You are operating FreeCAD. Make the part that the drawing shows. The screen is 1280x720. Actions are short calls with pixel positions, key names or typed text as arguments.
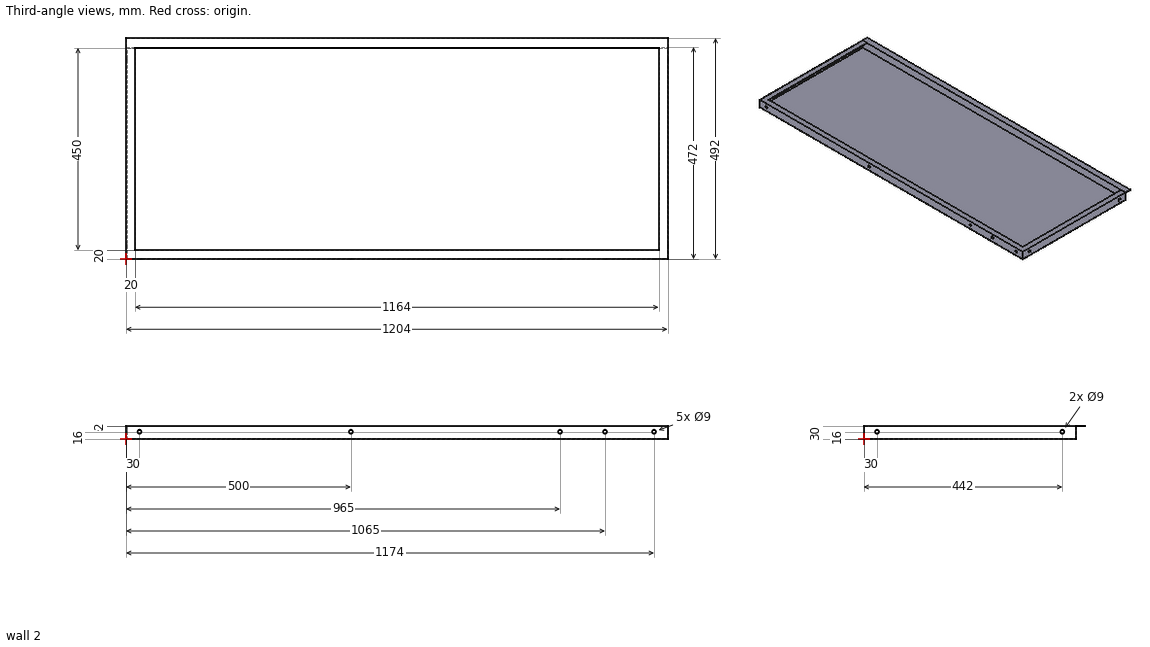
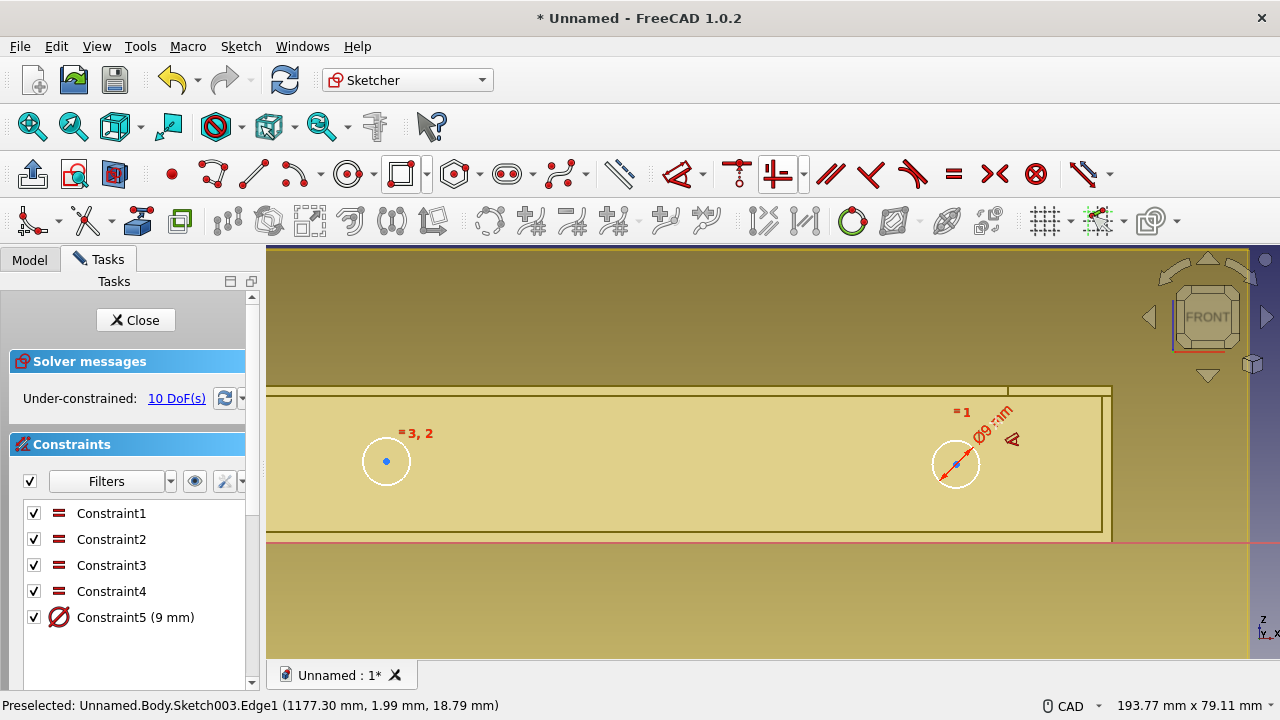
click(956, 464)
click(990, 503)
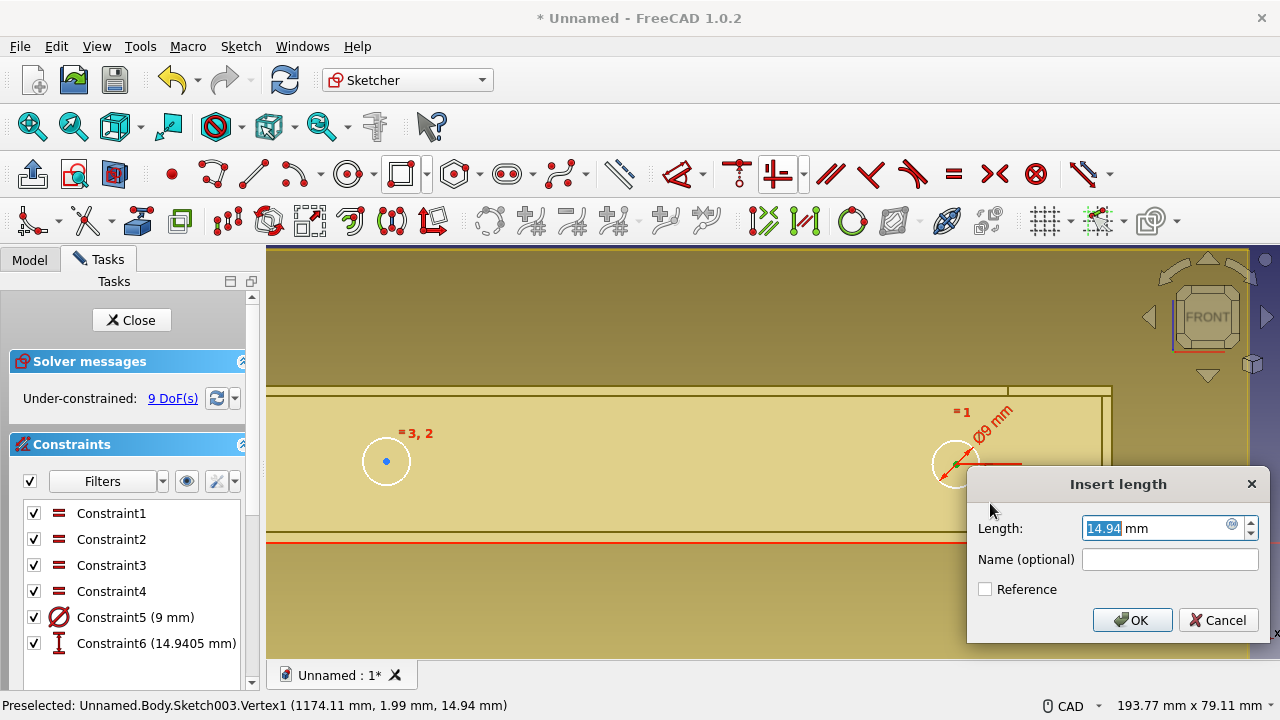
text(16)
key(Return)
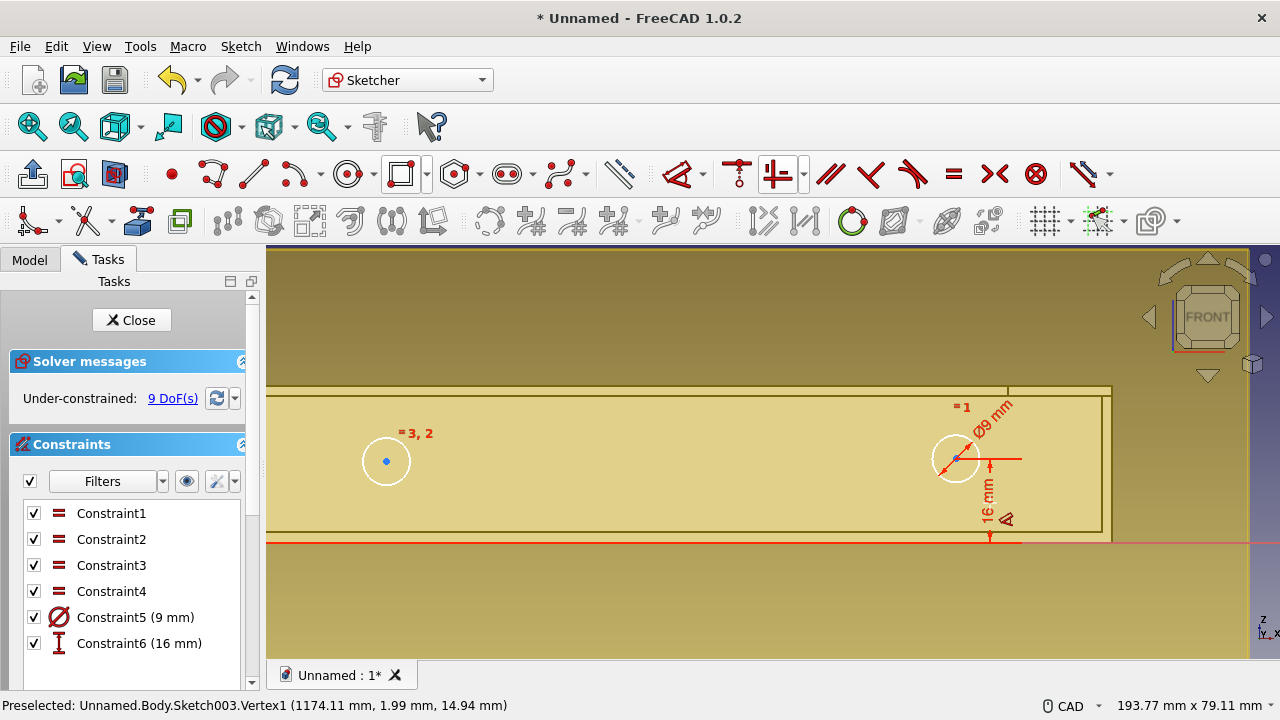
scroll(985, 448, down, 12)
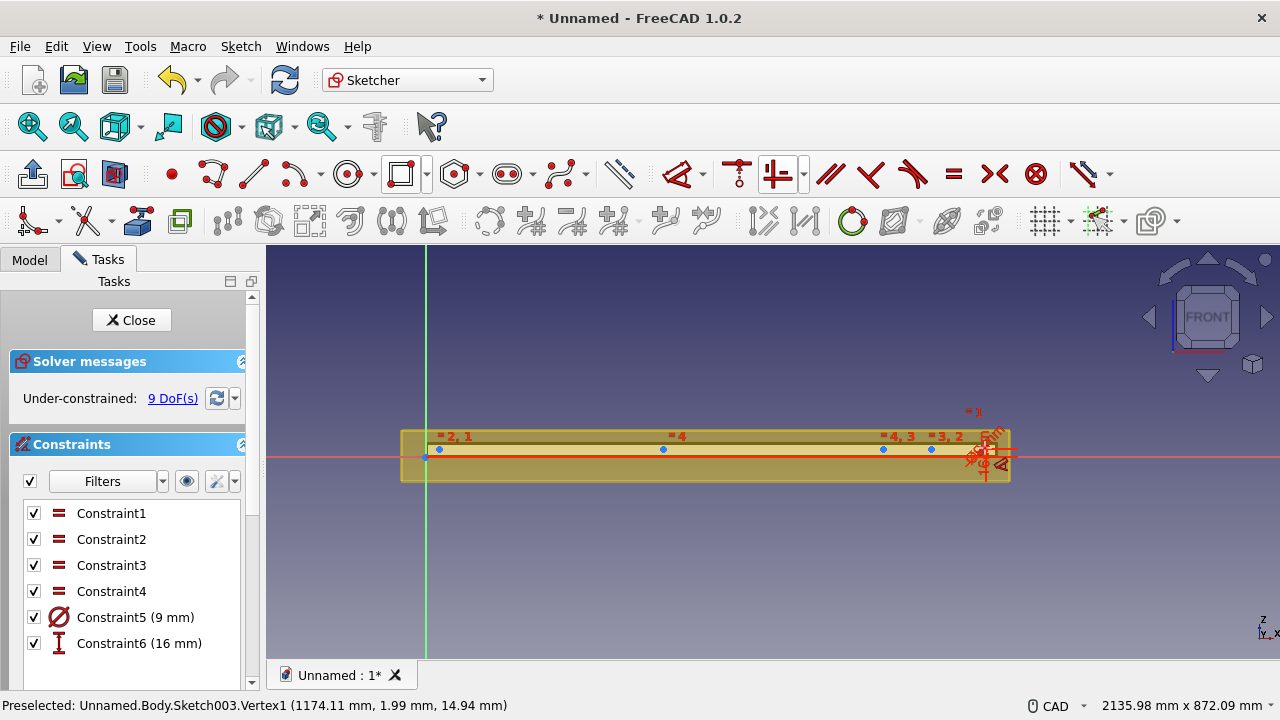
scroll(440, 450, up, 6)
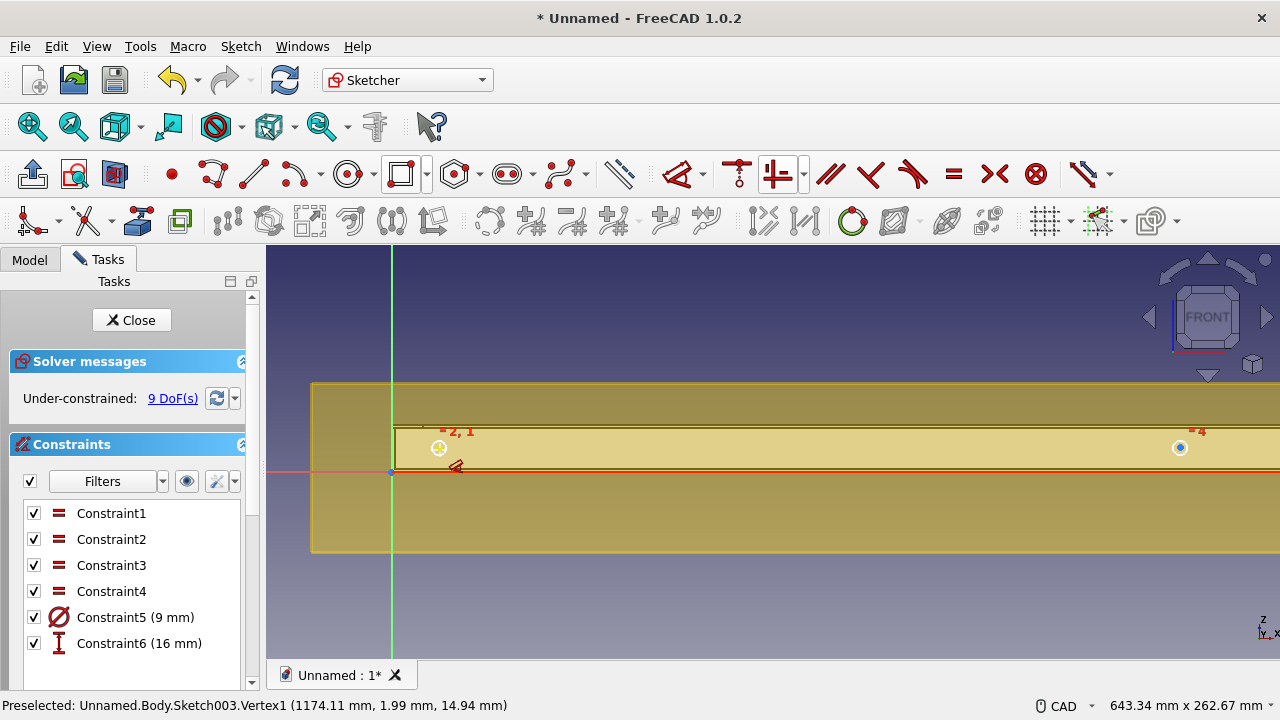
click(439, 448)
click(416, 506)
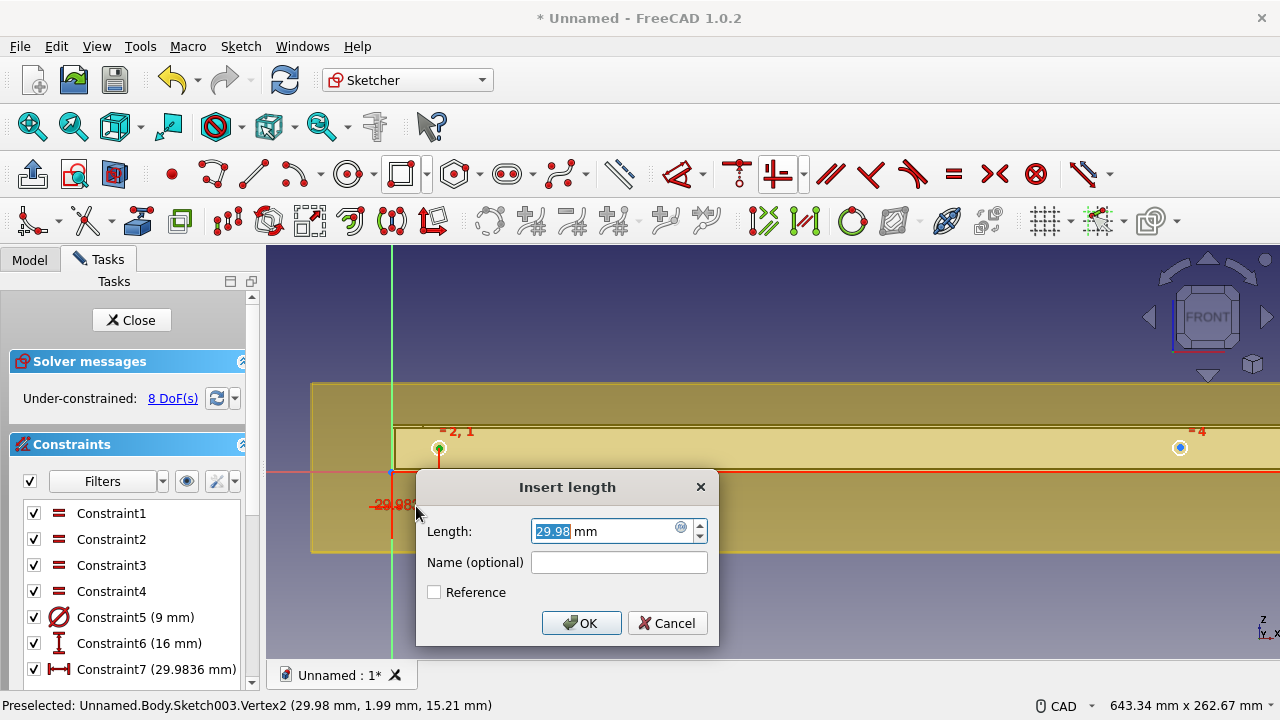
text(30)
key(Return)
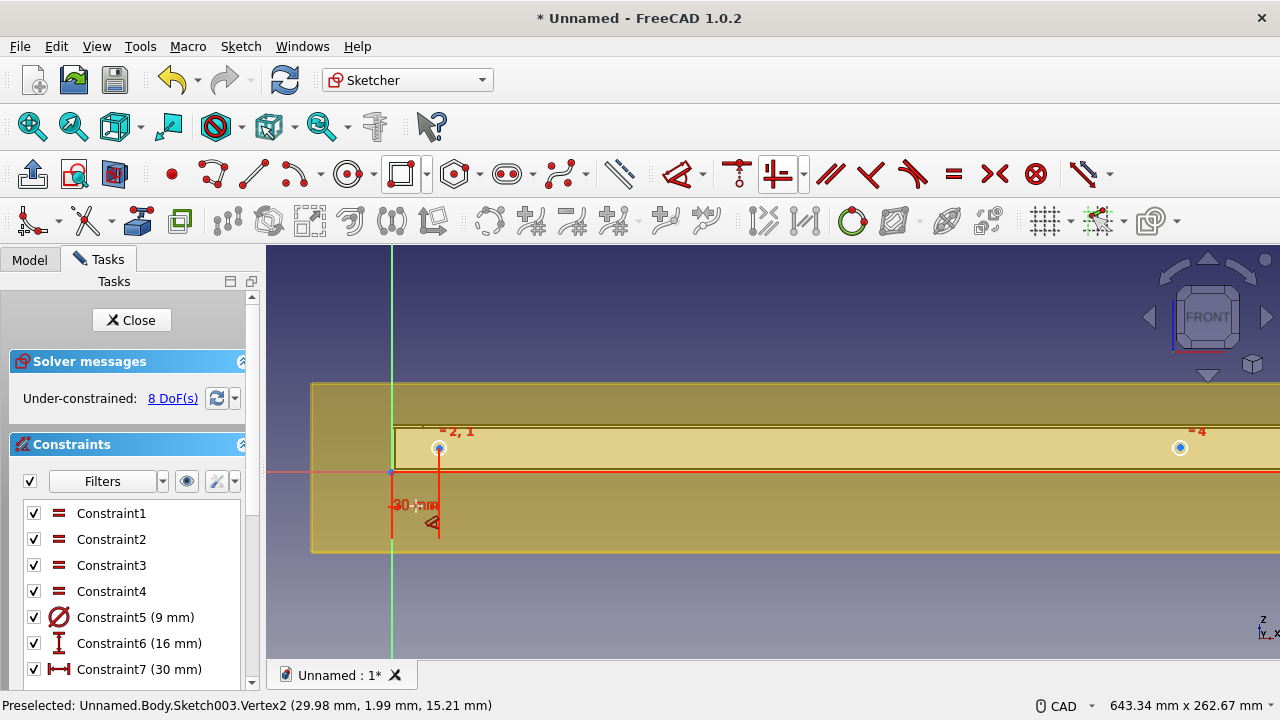
scroll(439, 448, up, 3)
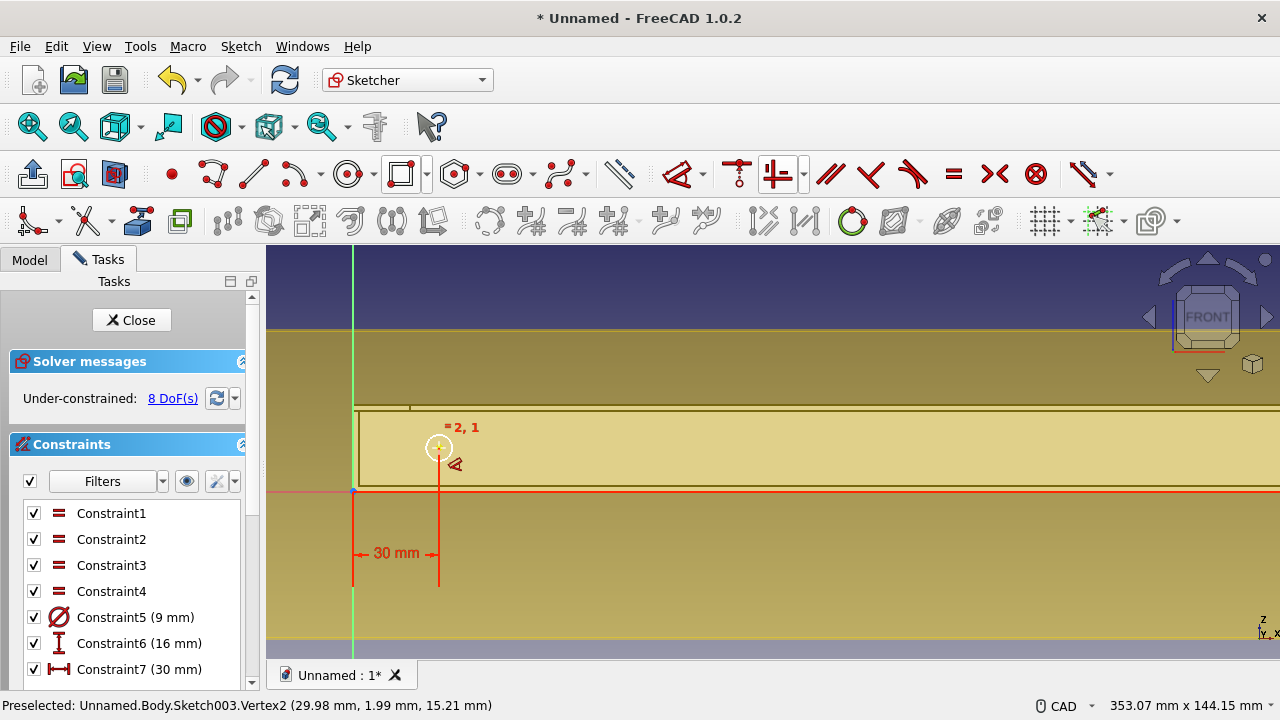
click(439, 448)
click(319, 470)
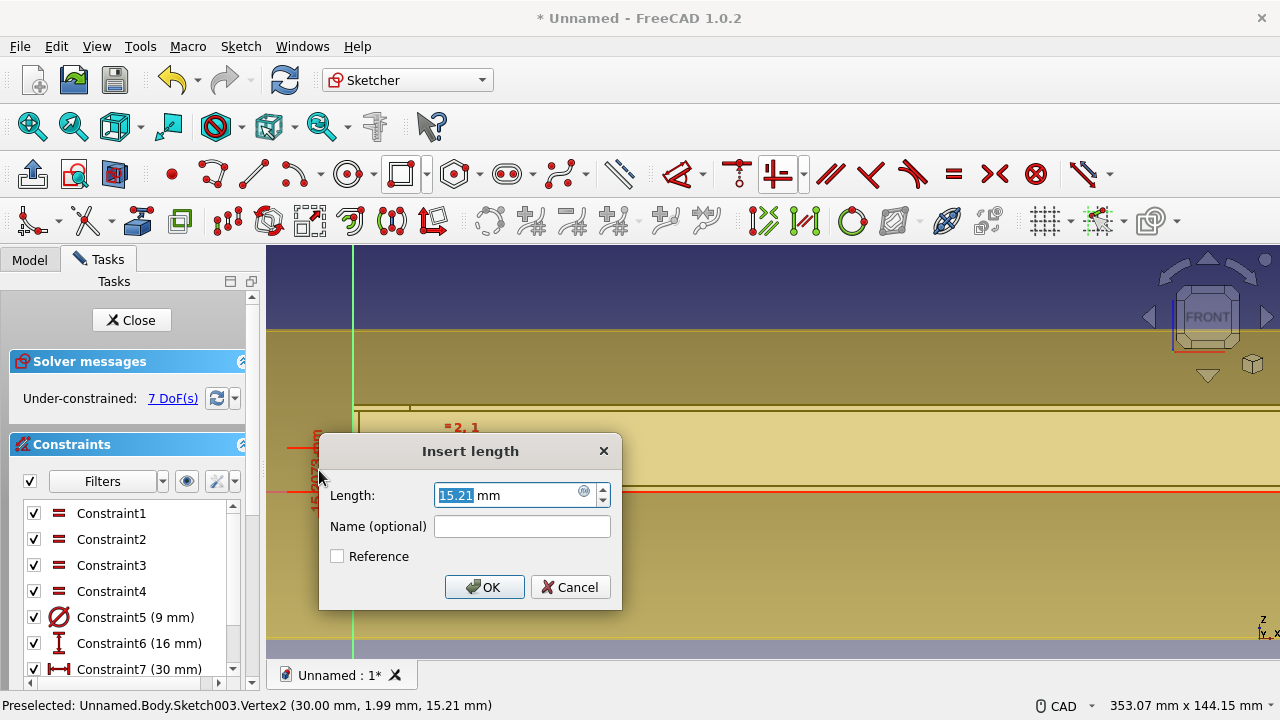
text(16)
key(Return)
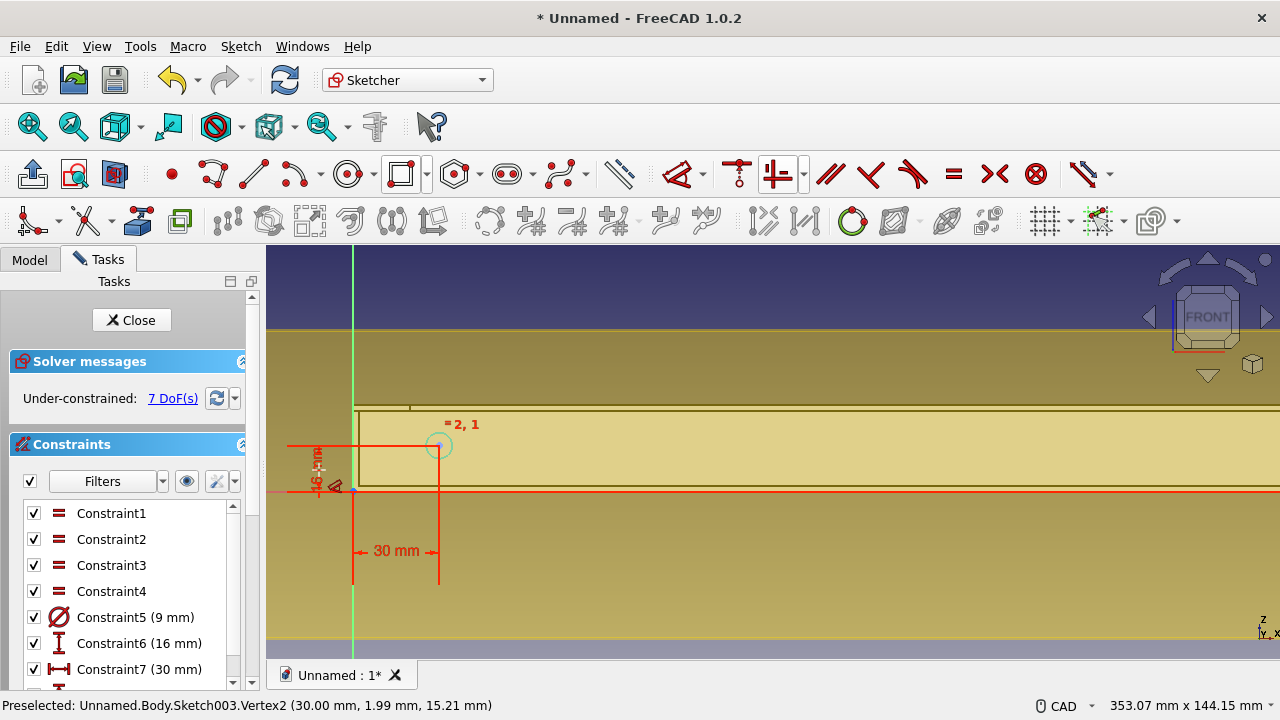
scroll(439, 450, down, 9)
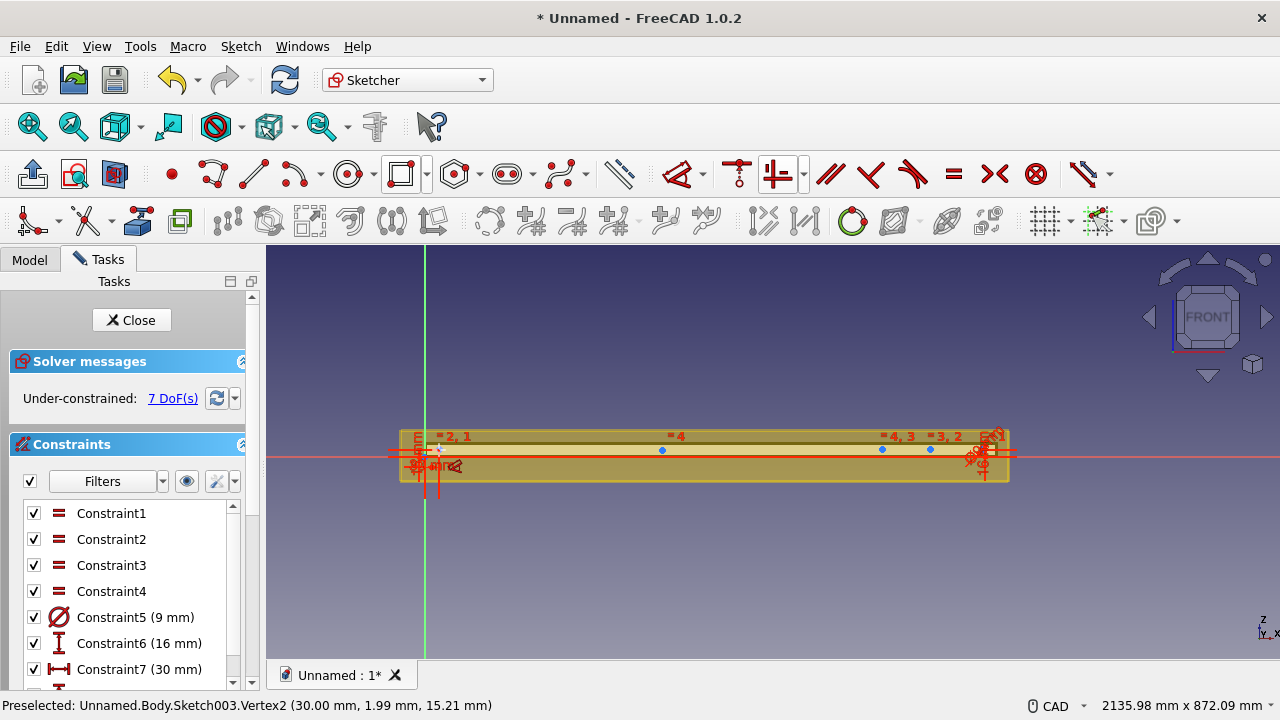
scroll(931, 450, up, 9)